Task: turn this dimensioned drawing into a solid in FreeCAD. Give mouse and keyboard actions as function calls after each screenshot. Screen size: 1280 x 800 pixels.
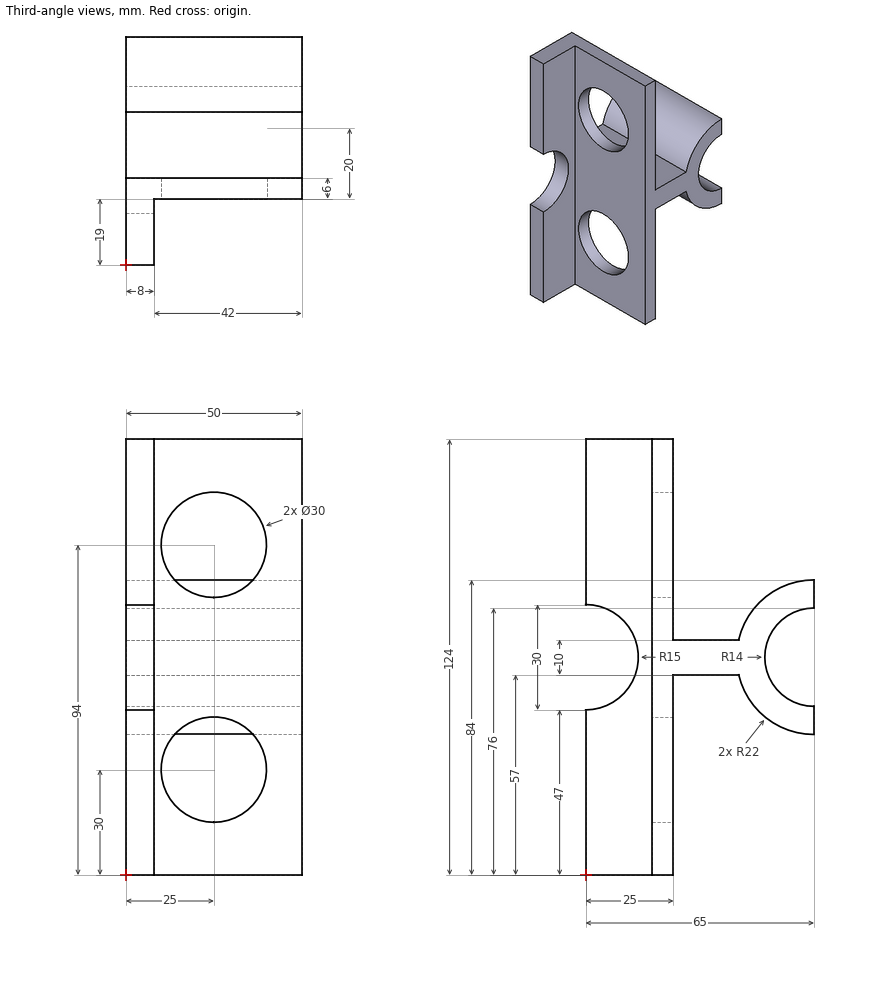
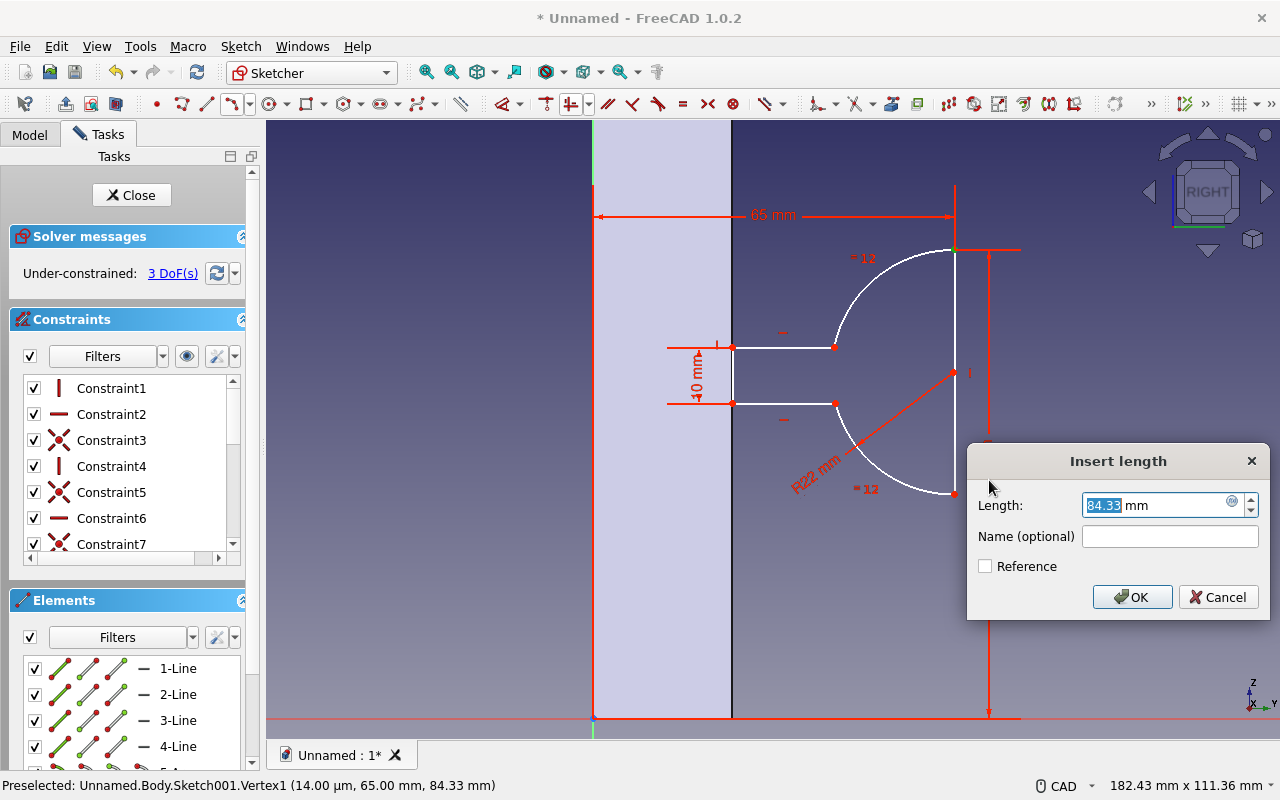
text(84)
key(Return)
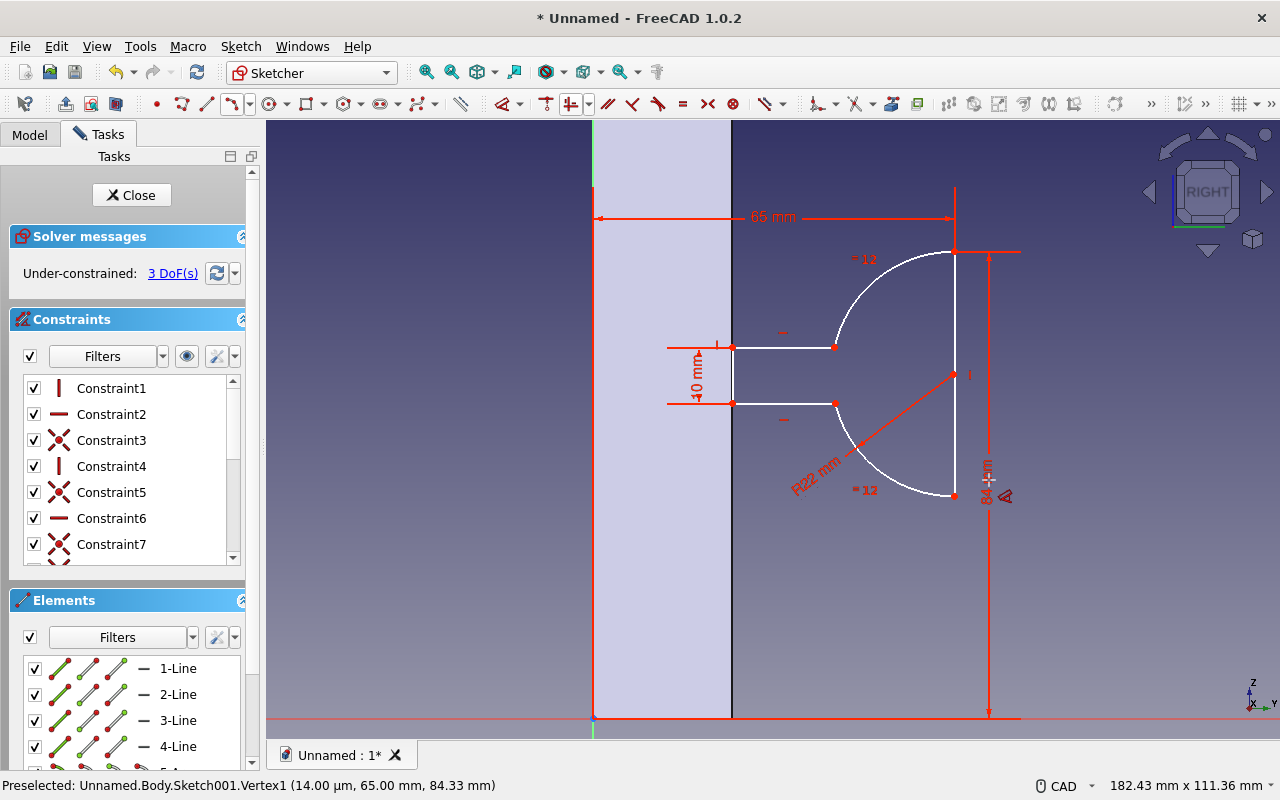
click(835, 404)
click(559, 557)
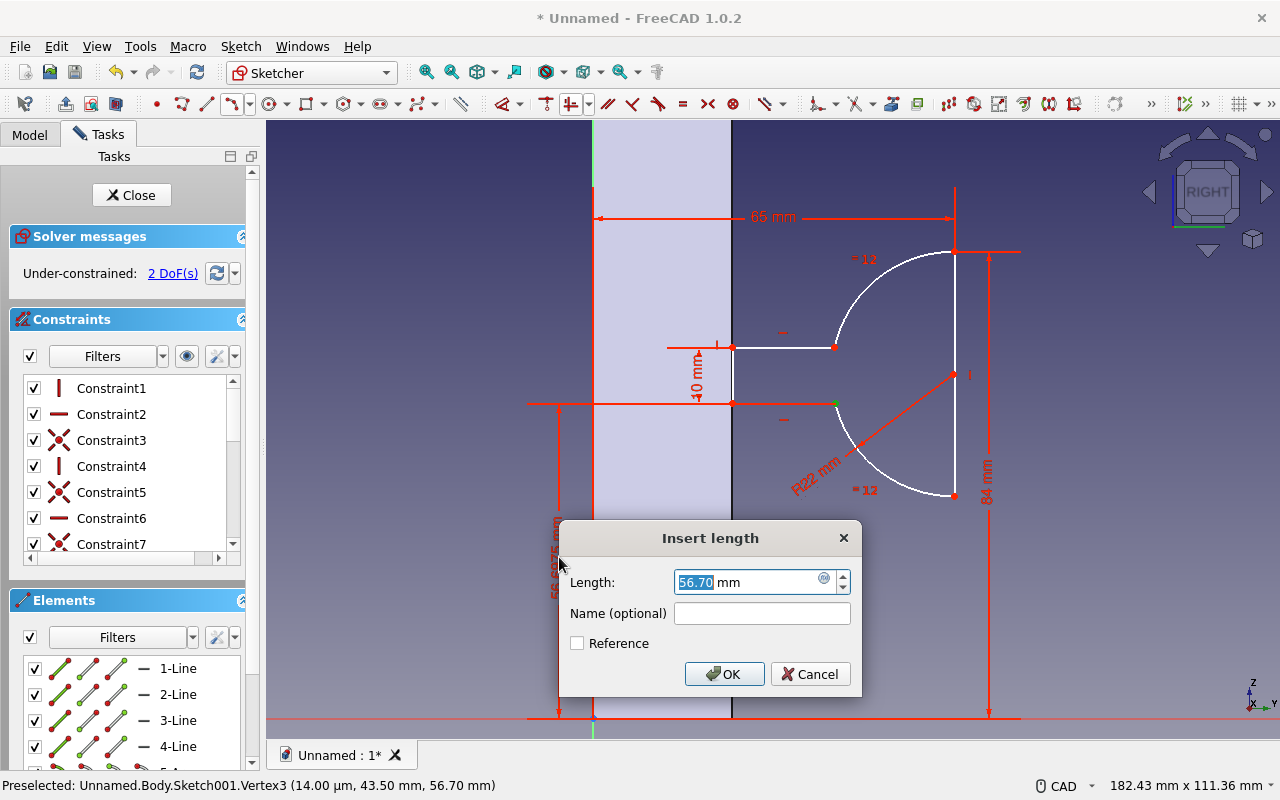
text(57)
key(Return)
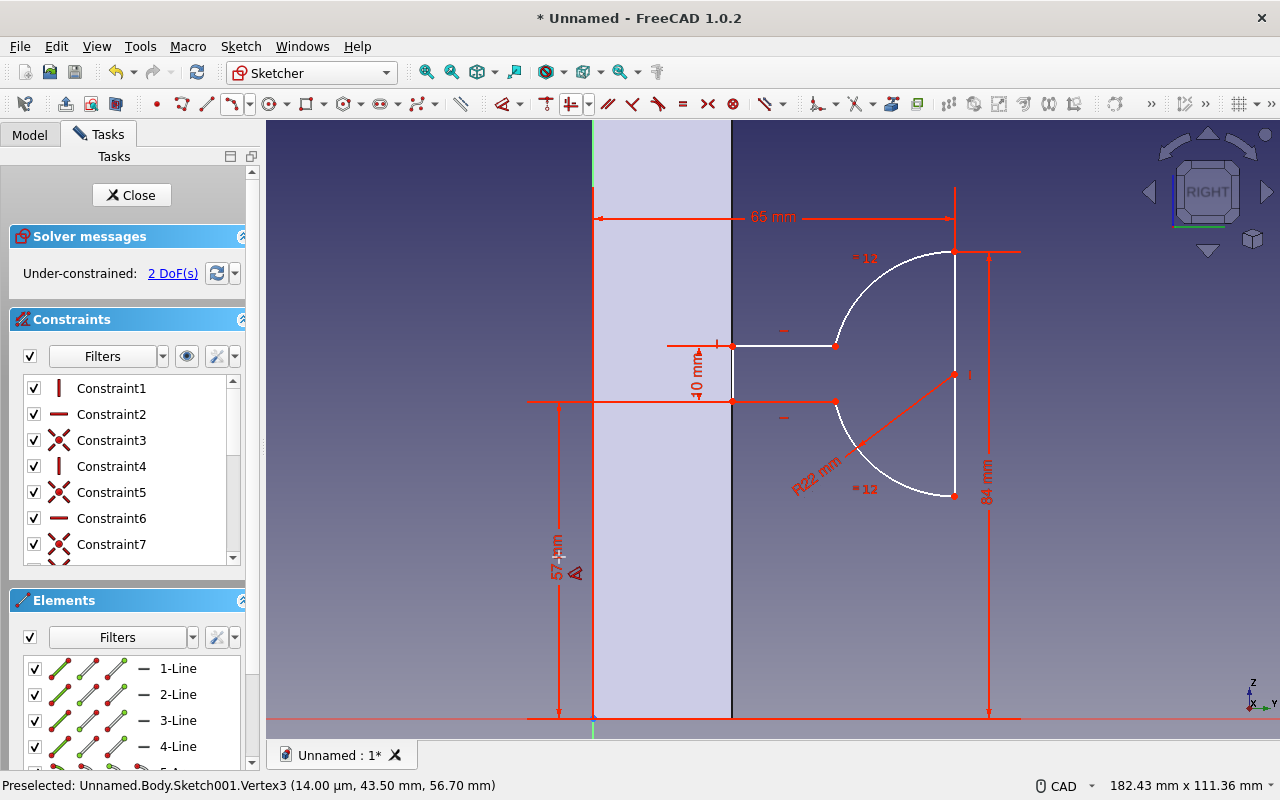
click(733, 402)
click(614, 368)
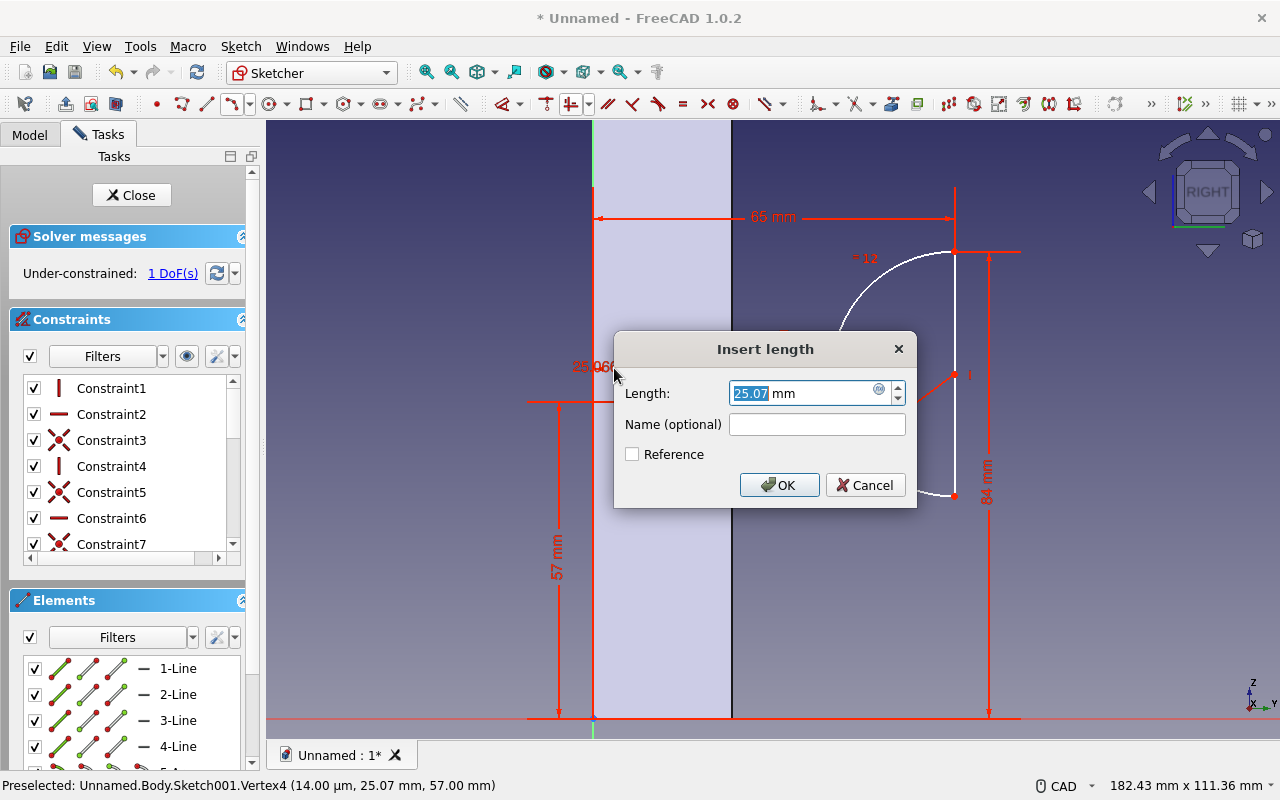
text(25)
key(Return)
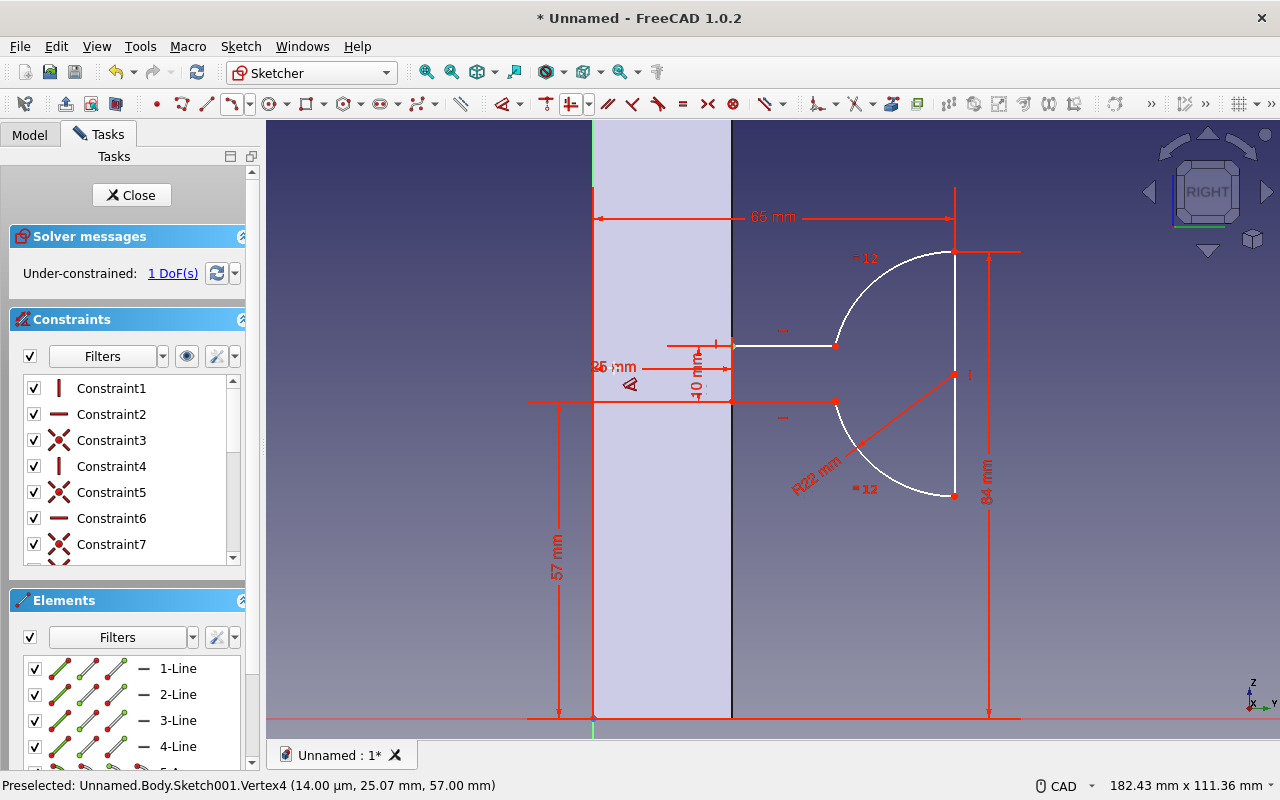
click(954, 374)
click(691, 340)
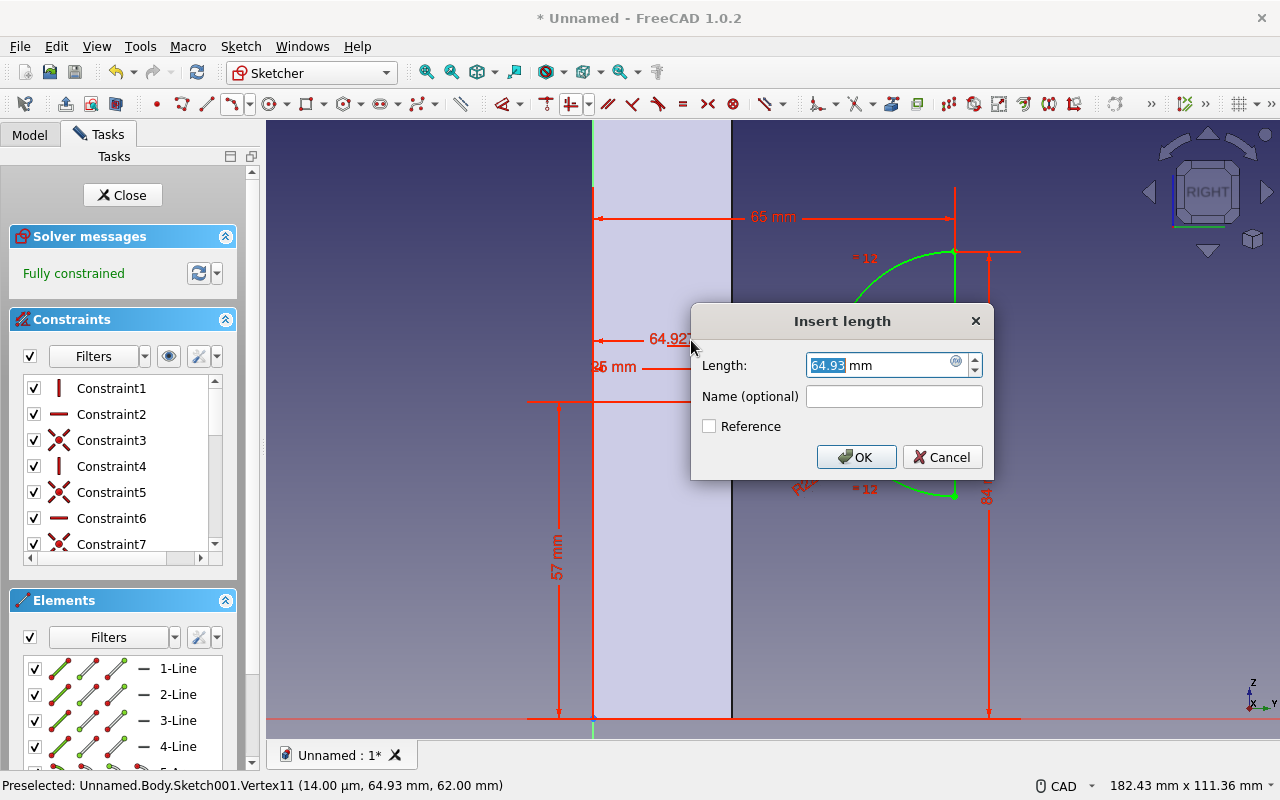
text(65)
key(Return)
key(Escape)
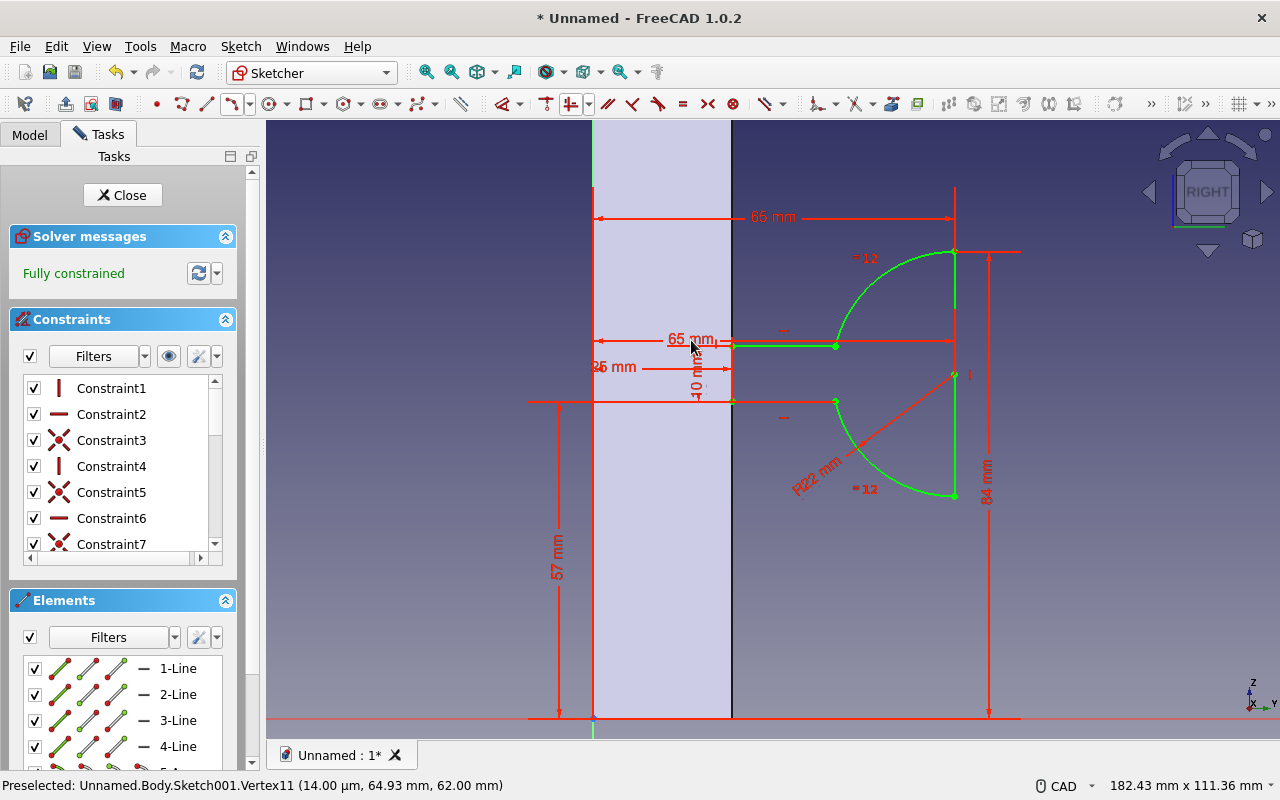
click(123, 195)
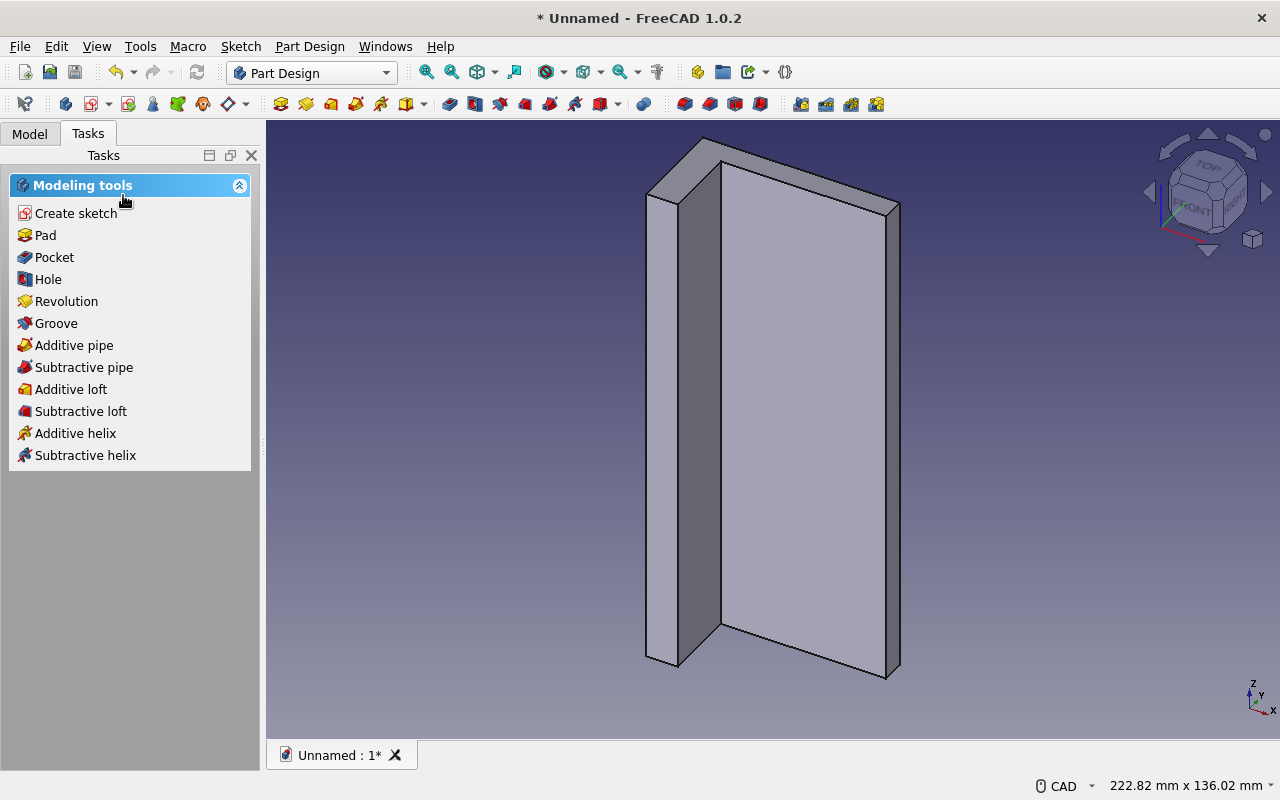
click(281, 104)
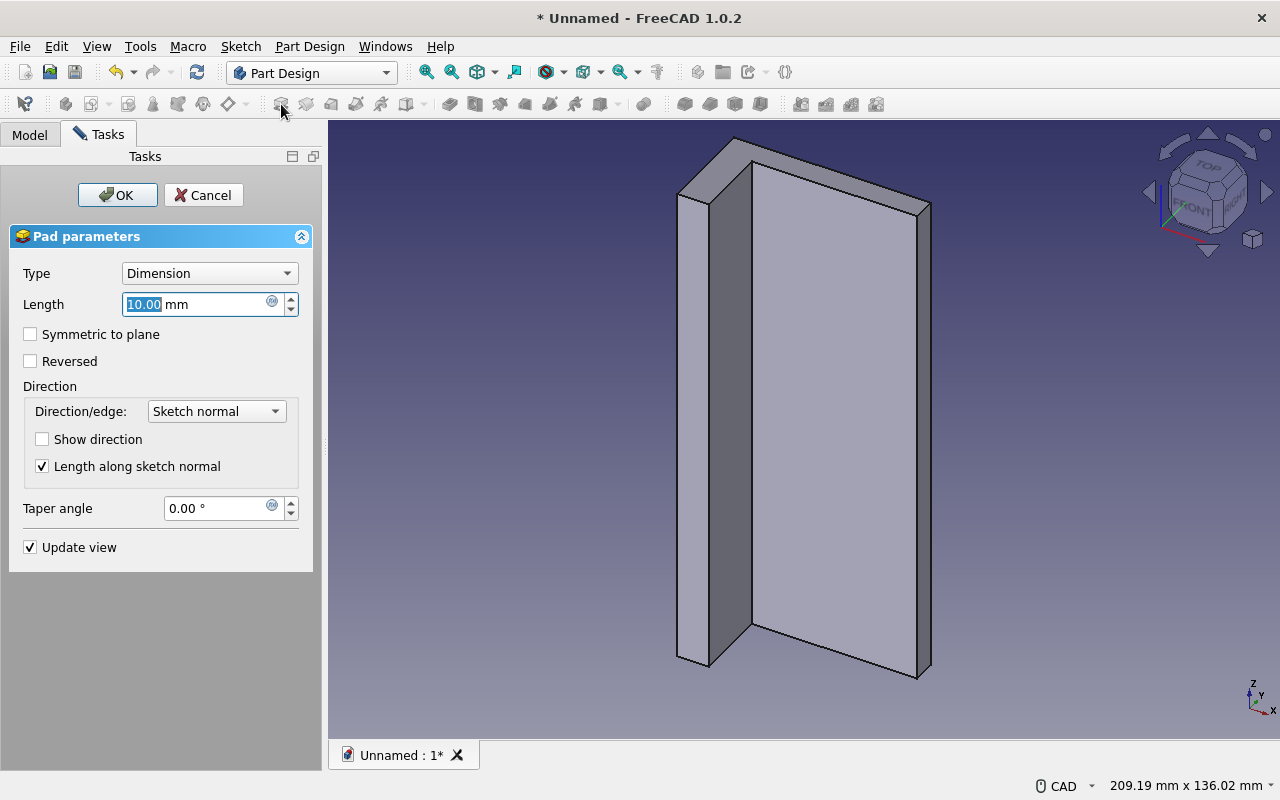
text(50)
key(Tab)